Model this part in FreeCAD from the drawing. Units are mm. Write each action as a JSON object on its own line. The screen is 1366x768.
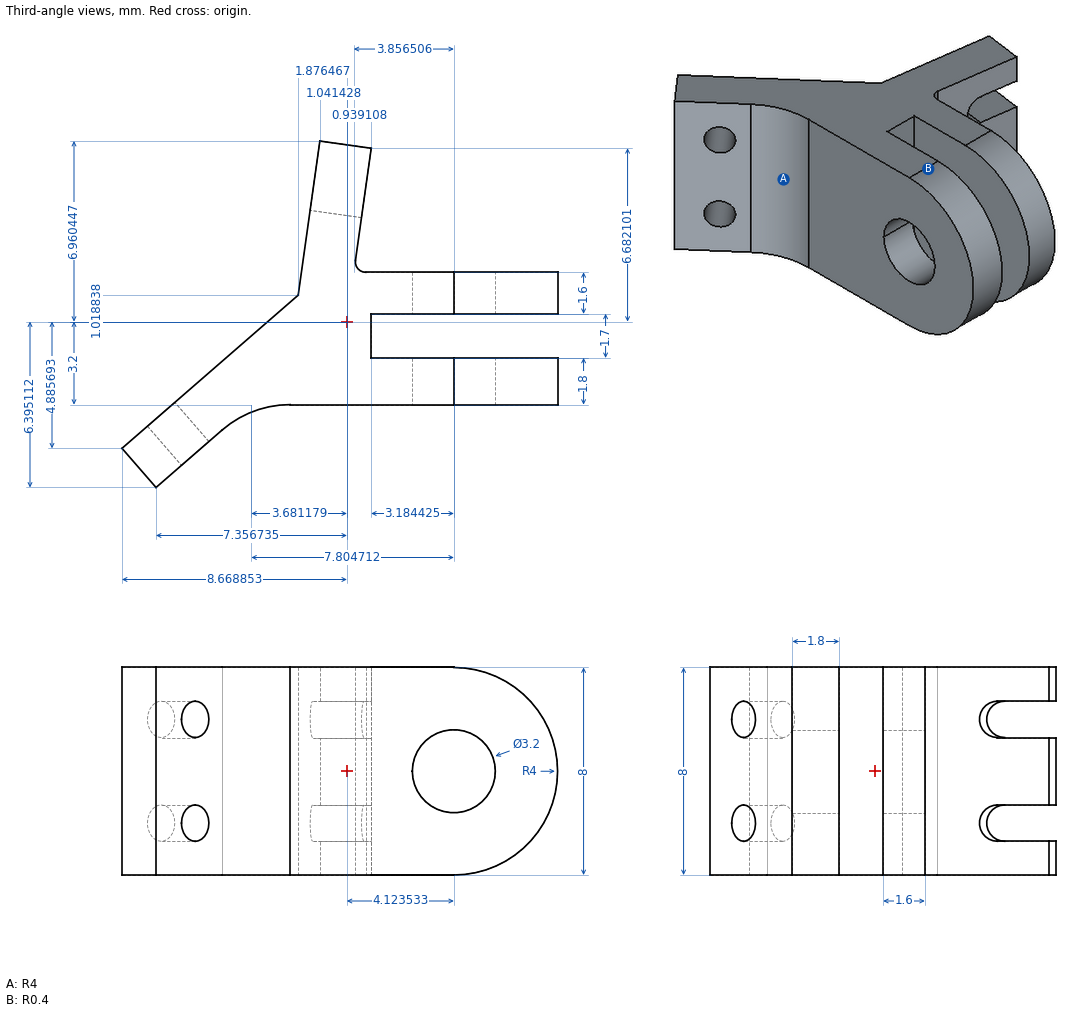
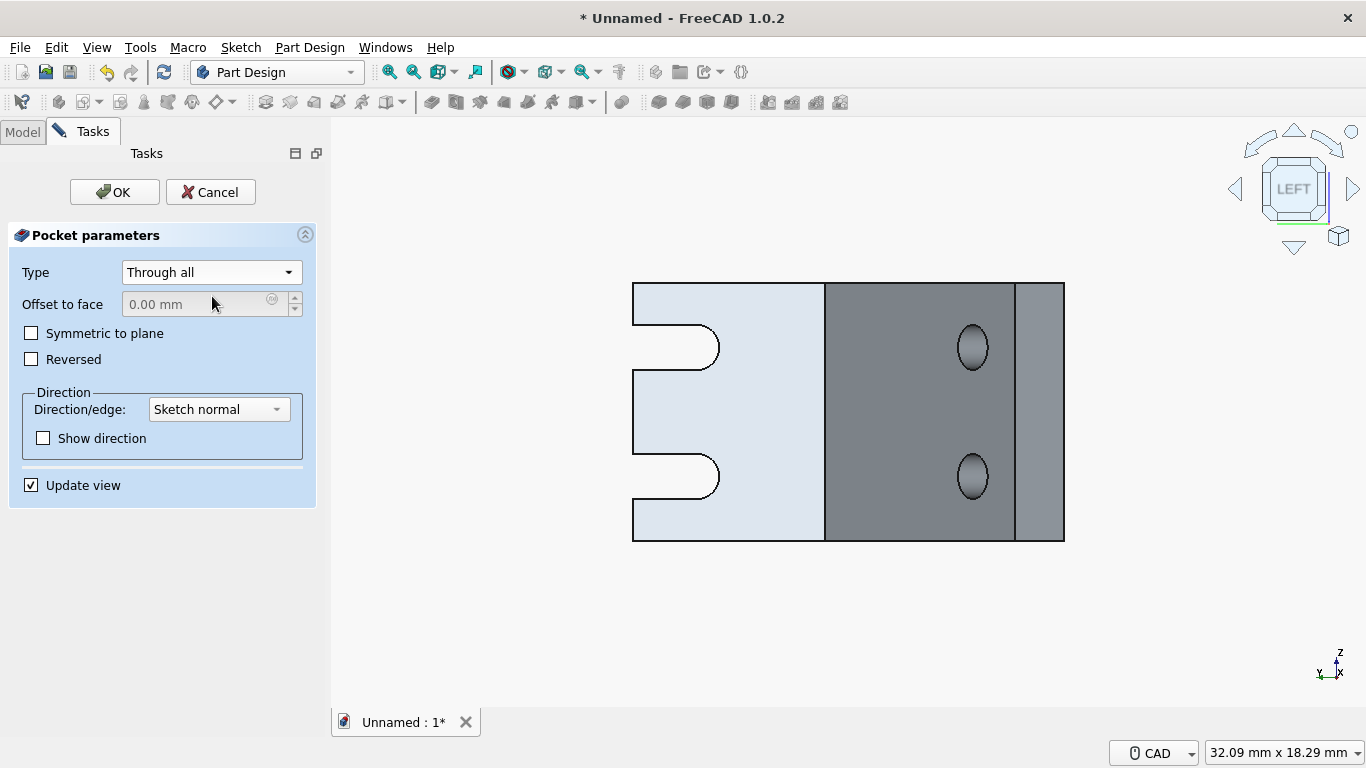
{"action": "left_click", "coordinate": [115, 192]}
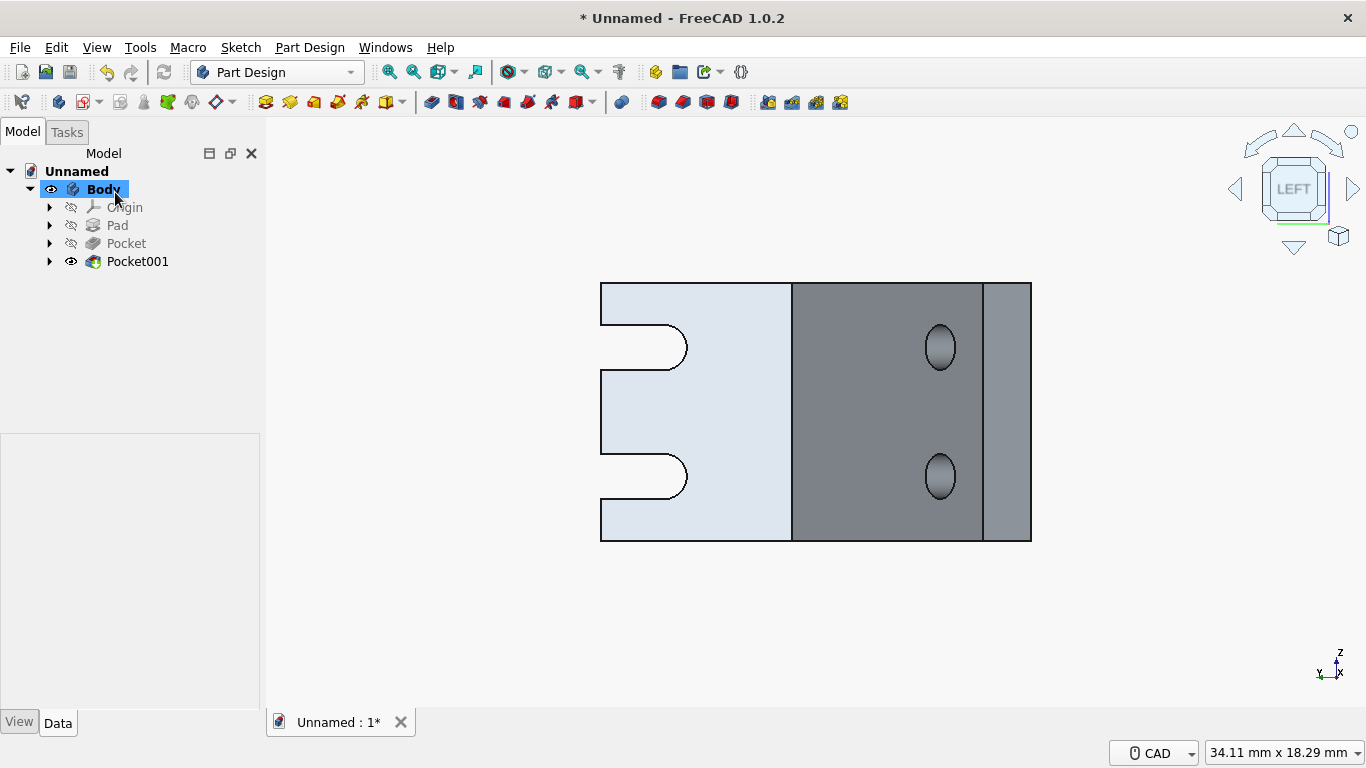
{"action": "left_click", "coordinate": [390, 72]}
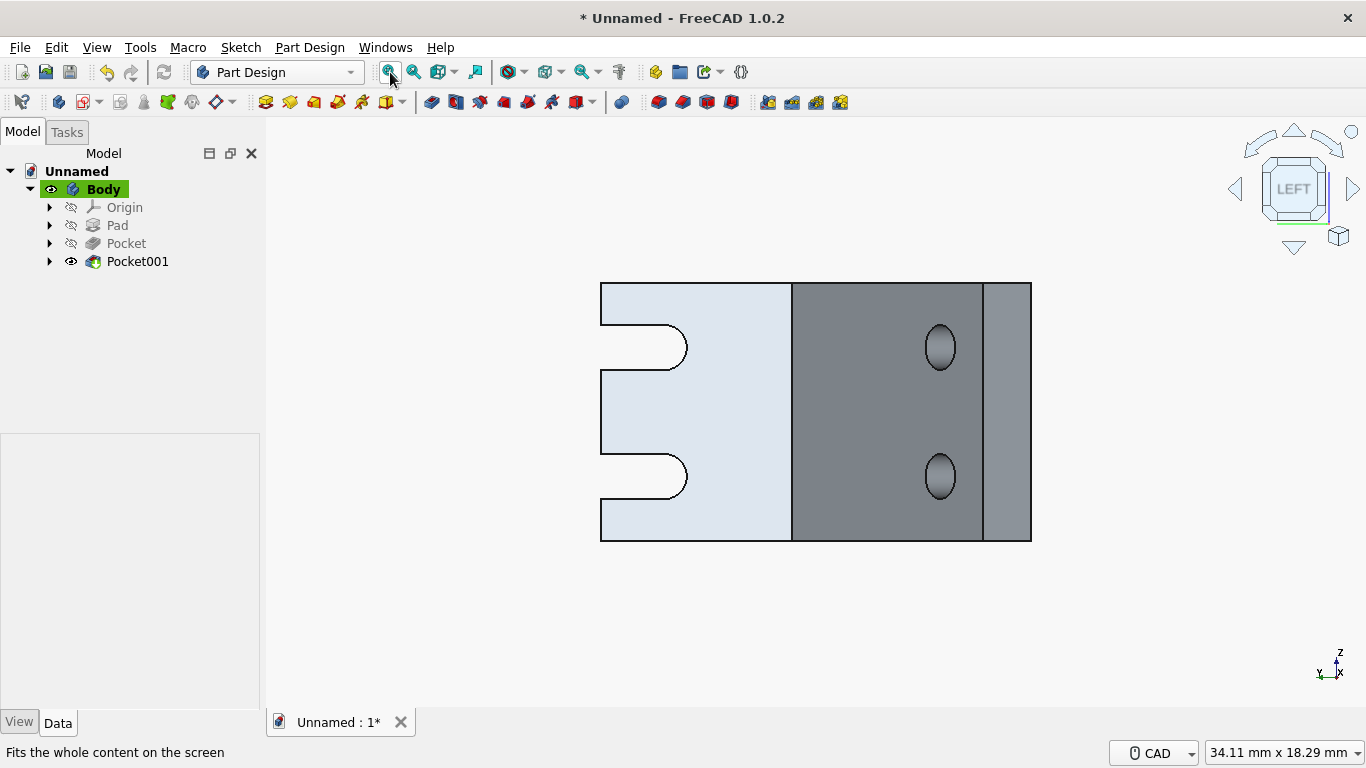
{"action": "left_click", "coordinate": [84, 102]}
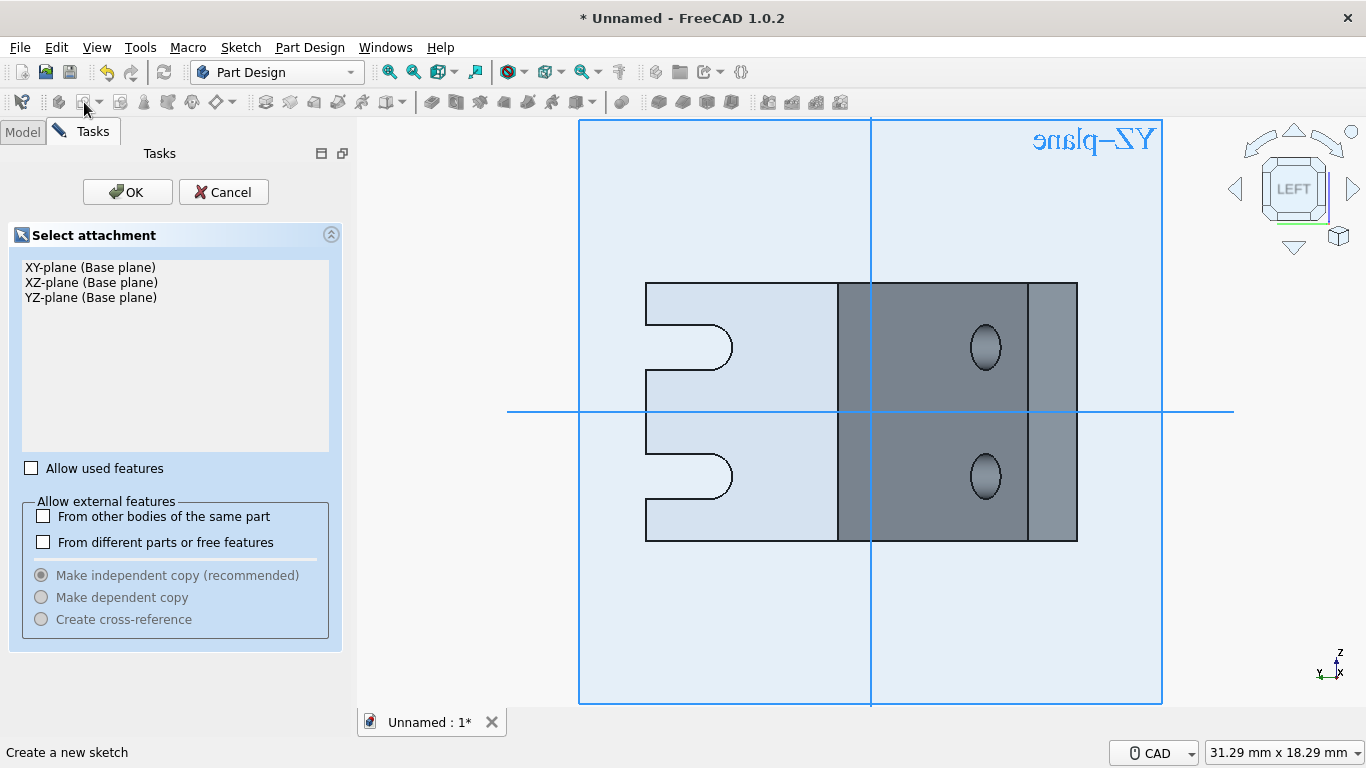
{"action": "left_click", "coordinate": [82, 268]}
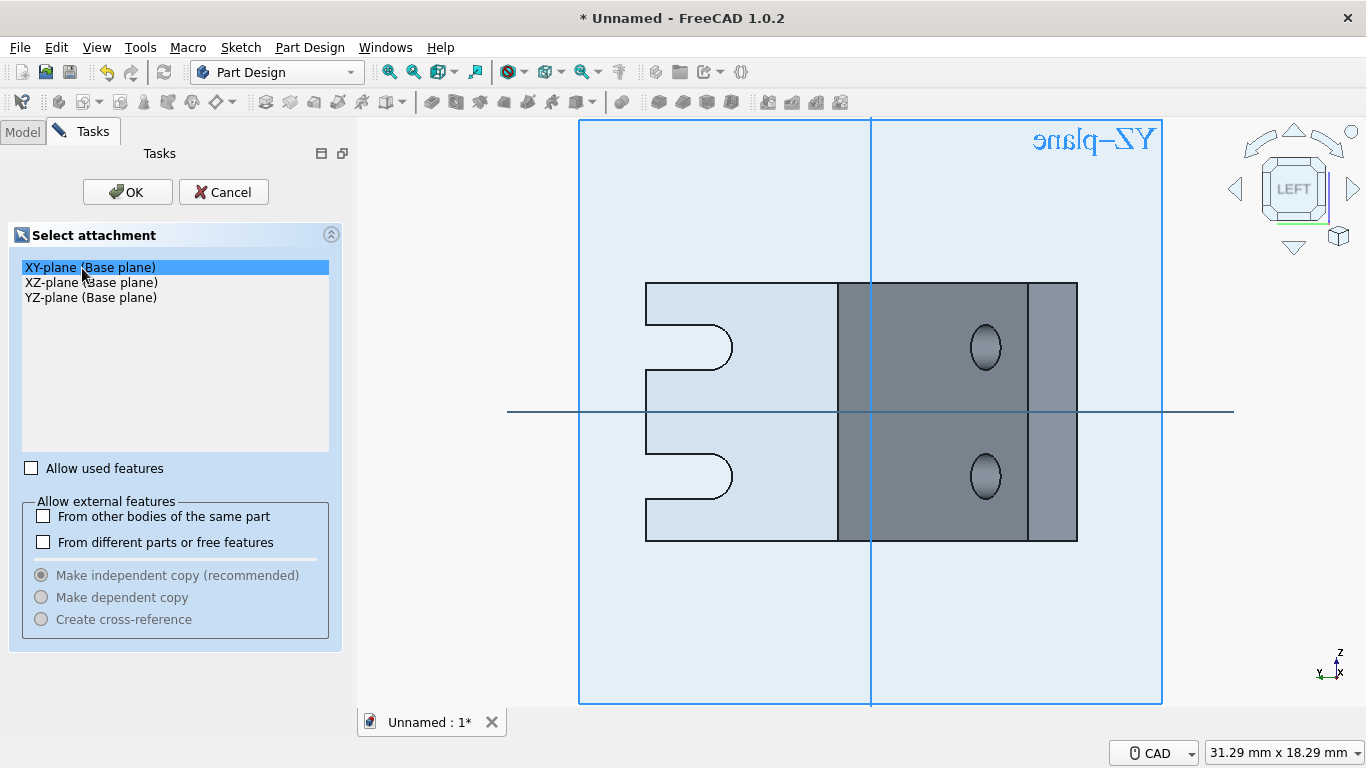
{"action": "left_click", "coordinate": [128, 192]}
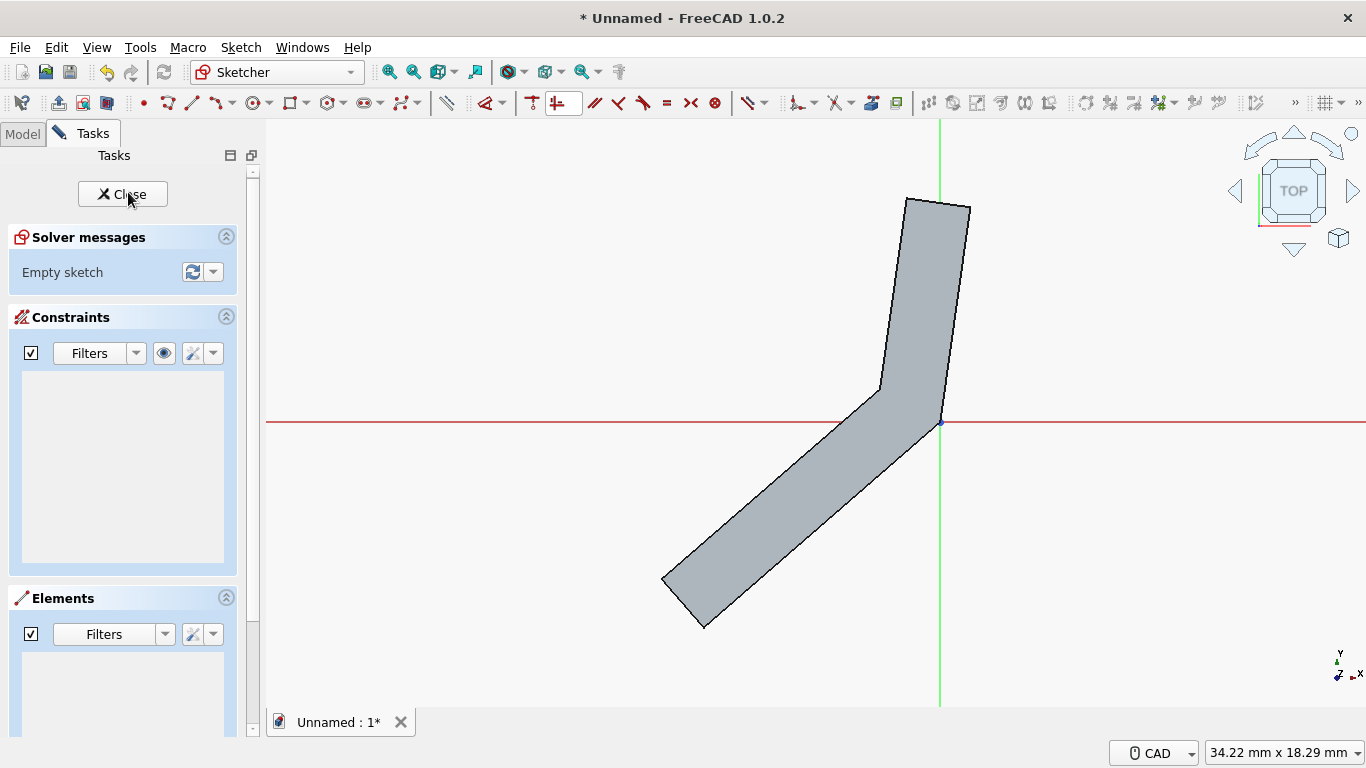
{"action": "left_click", "coordinate": [108, 104]}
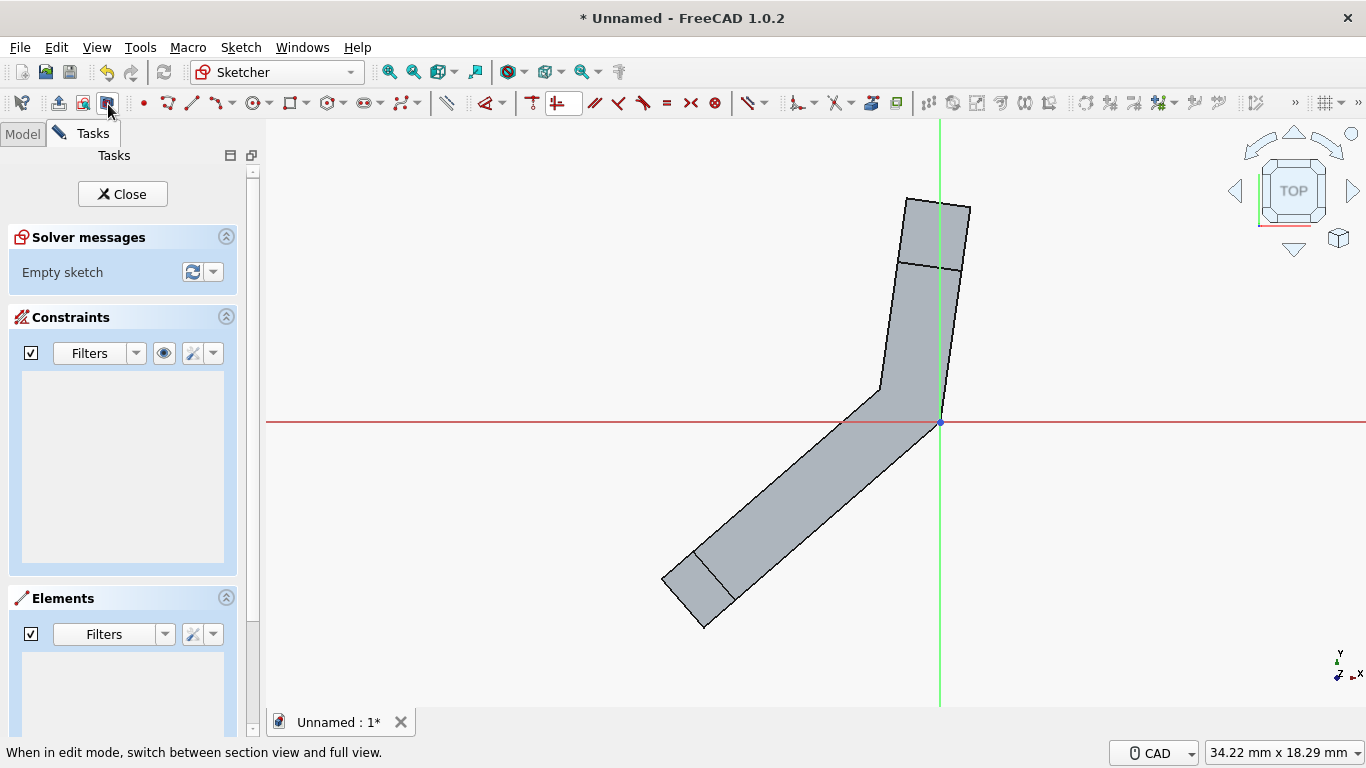
{"action": "scroll", "coordinate": [1110, 467], "scroll_direction": "up", "scroll_amount": 4}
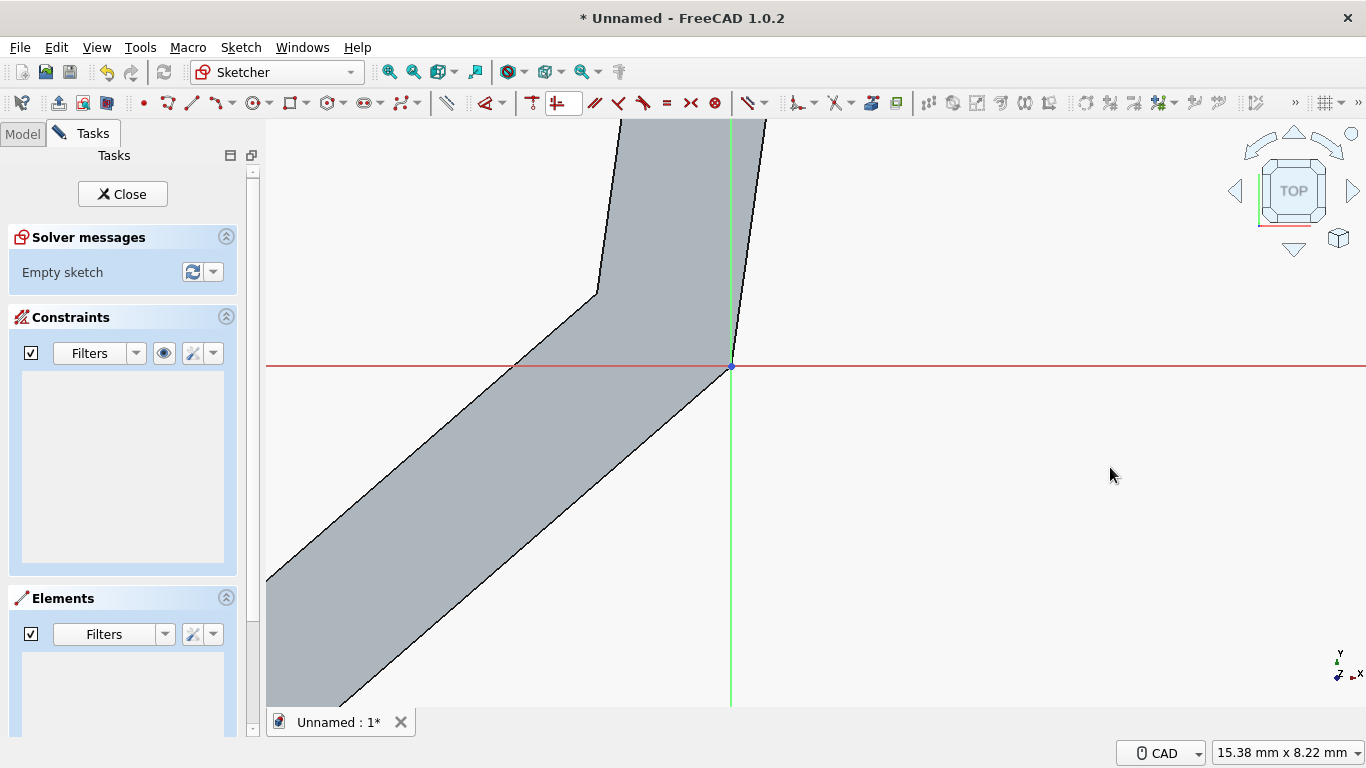
{"action": "left_click", "coordinate": [168, 104]}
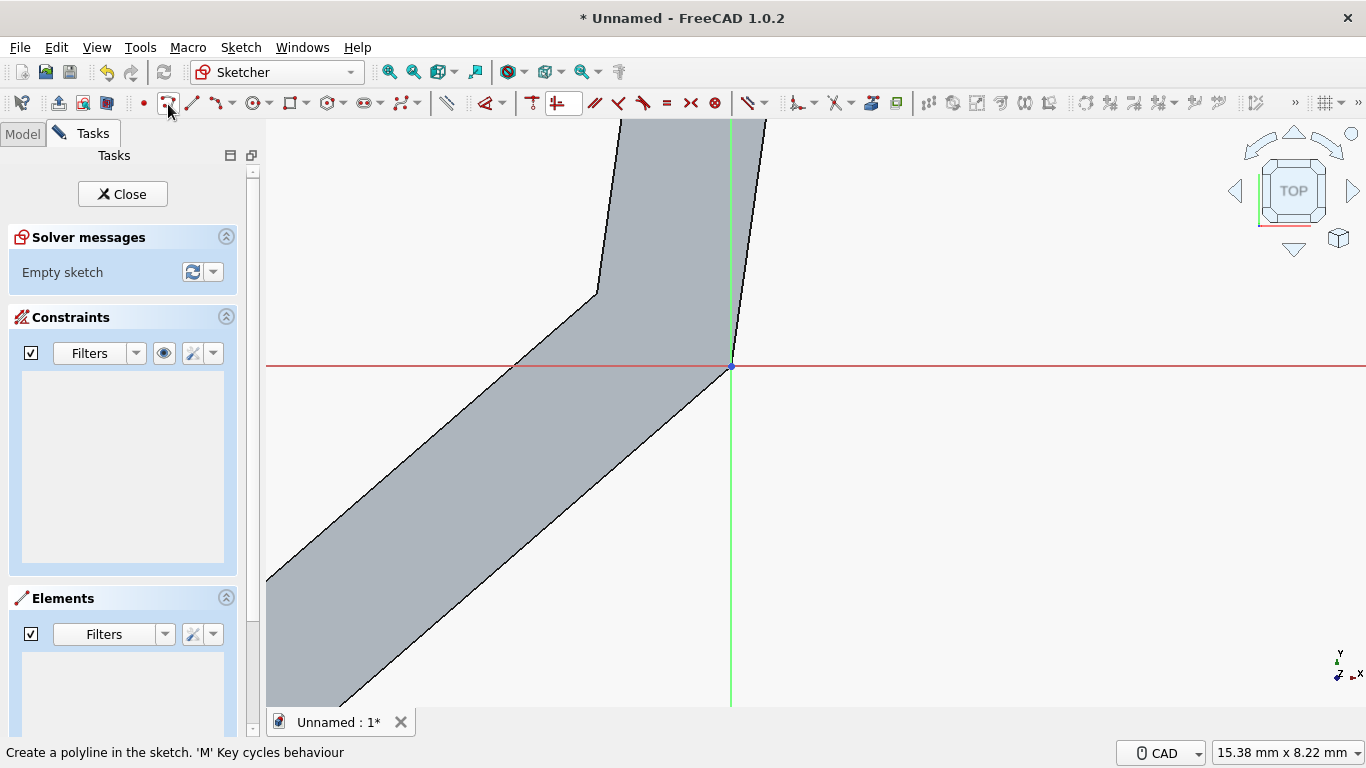
{"action": "left_click", "coordinate": [731, 366]}
{"action": "left_click", "coordinate": [468, 595]}
{"action": "left_click", "coordinate": [1026, 595]}
{"action": "left_click", "coordinate": [1026, 466]}
{"action": "left_click", "coordinate": [798, 466]}
{"action": "left_click", "coordinate": [798, 345]}
{"action": "left_click", "coordinate": [1026, 345]}
{"action": "left_click", "coordinate": [1026, 230]}
{"action": "left_click", "coordinate": [750, 230]}
{"action": "left_click", "coordinate": [731, 366]}
{"action": "key", "text": "Escape"}
{"action": "key", "text": "Escape"}